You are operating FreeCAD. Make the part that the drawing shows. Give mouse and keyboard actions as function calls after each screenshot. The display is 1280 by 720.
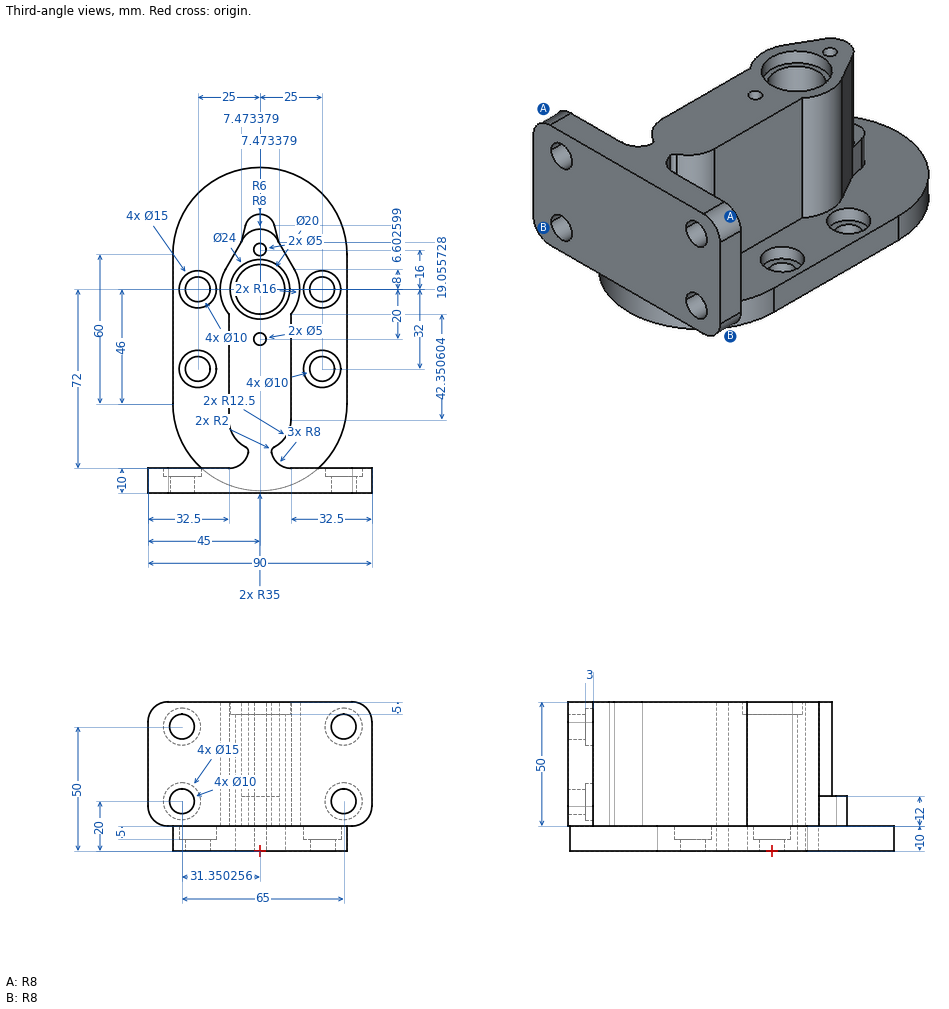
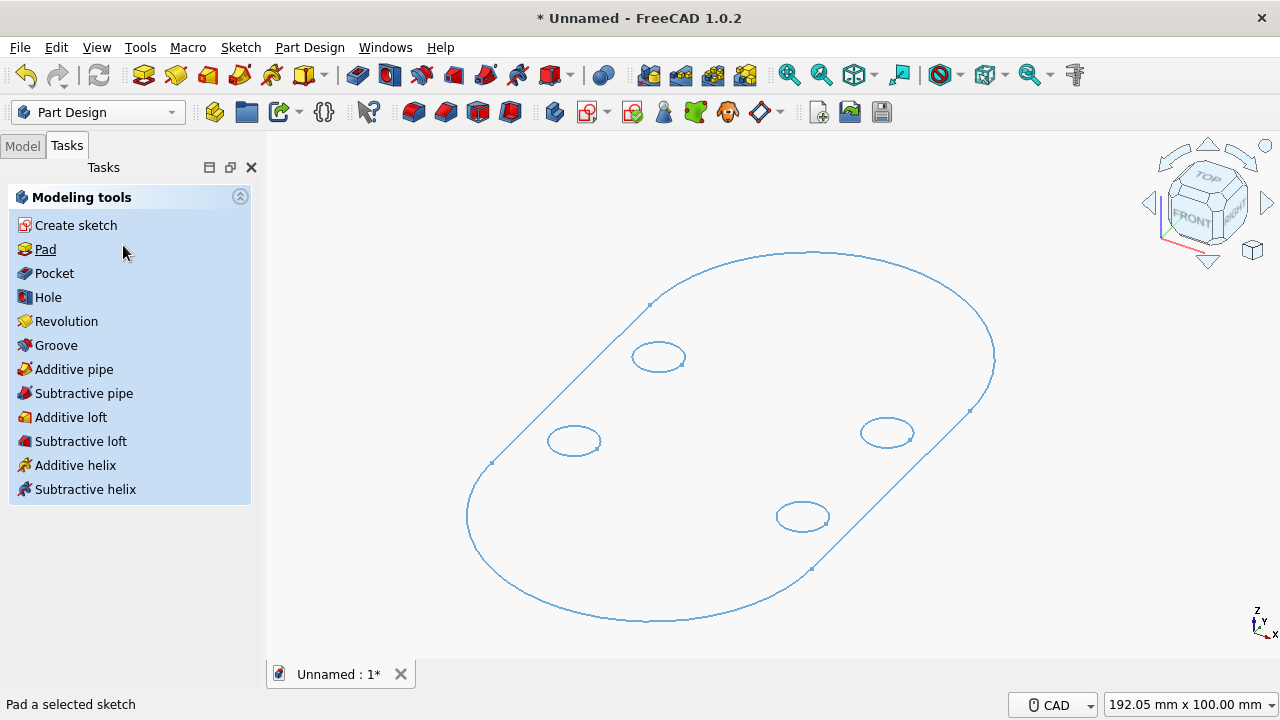
click(144, 76)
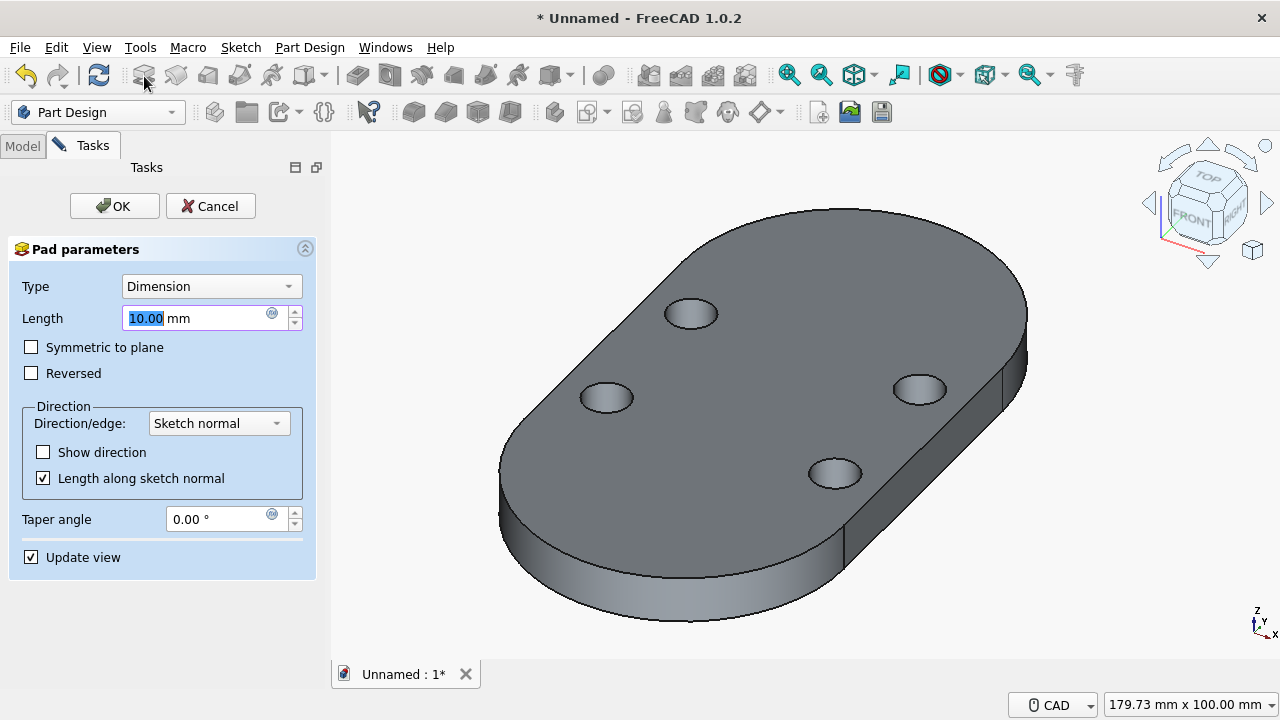
text(10)
key(Tab)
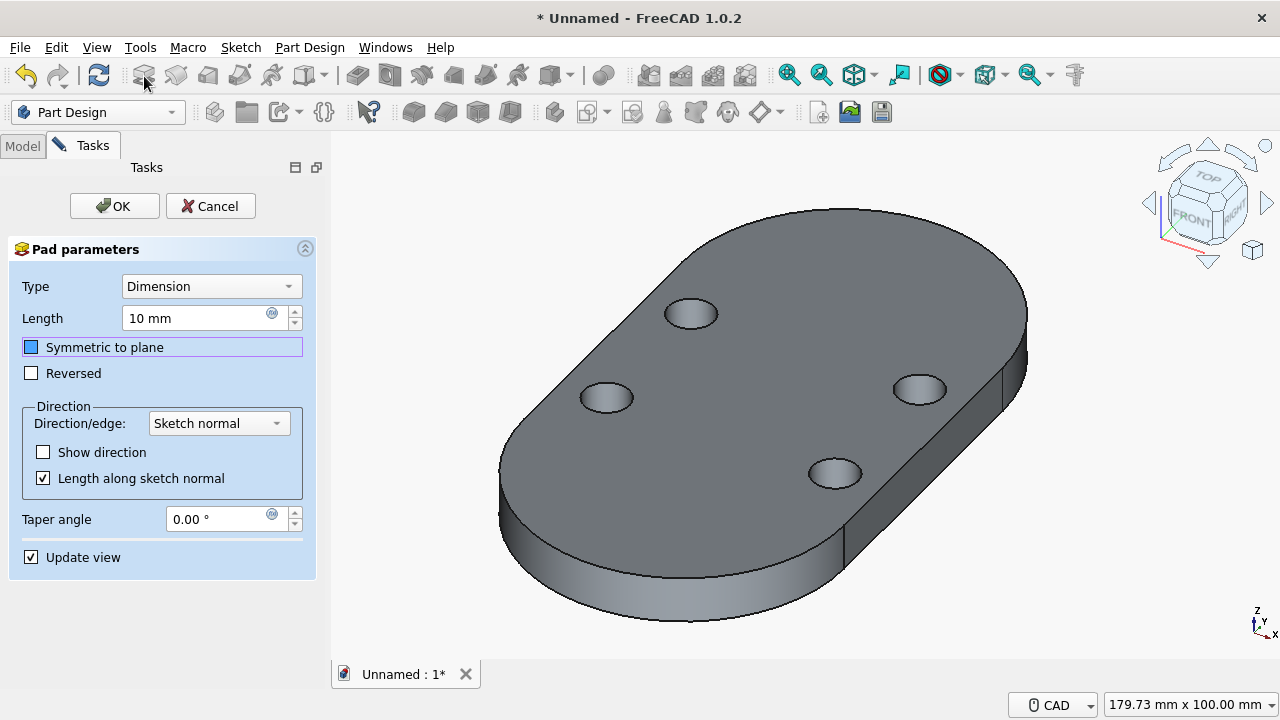
click(115, 206)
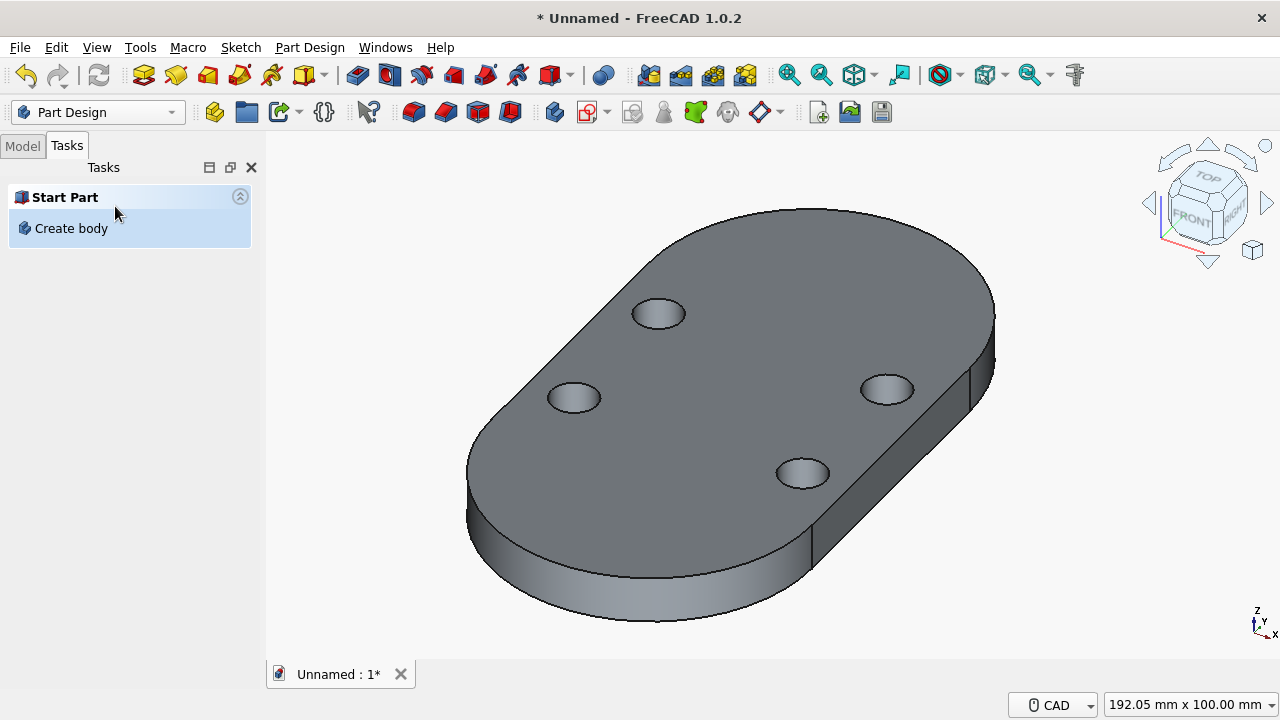
click(23, 145)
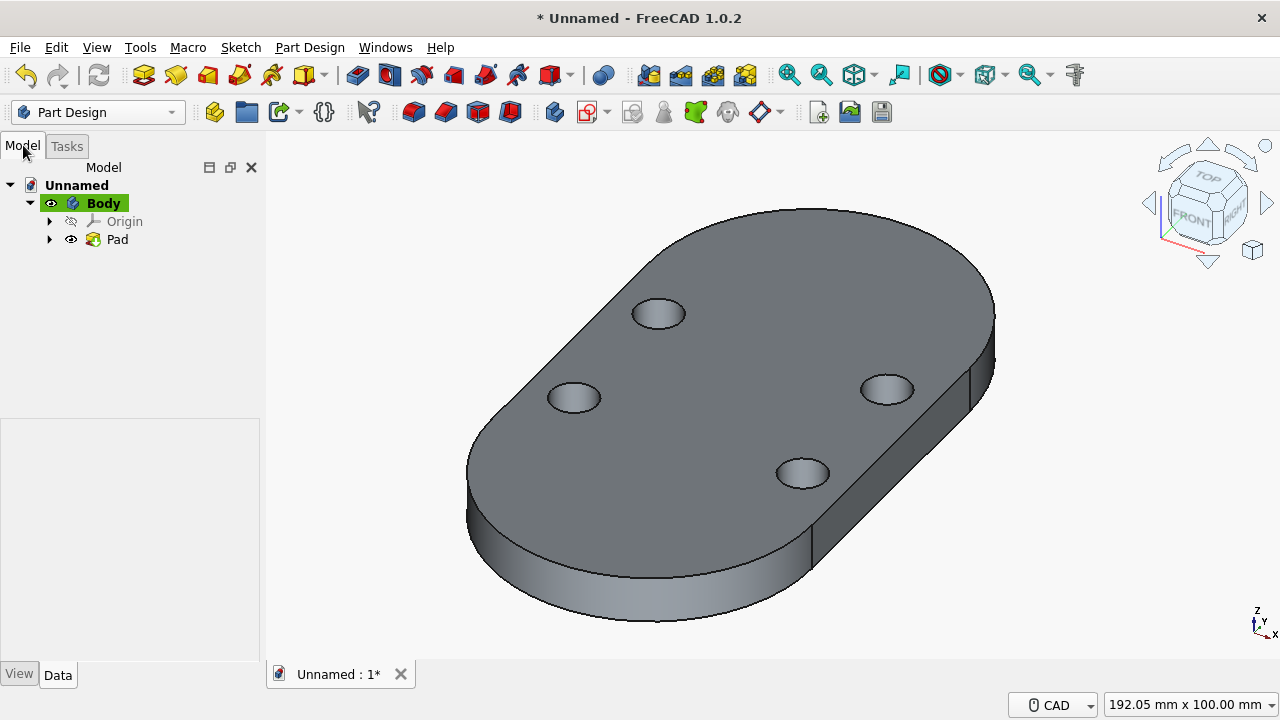
click(50, 221)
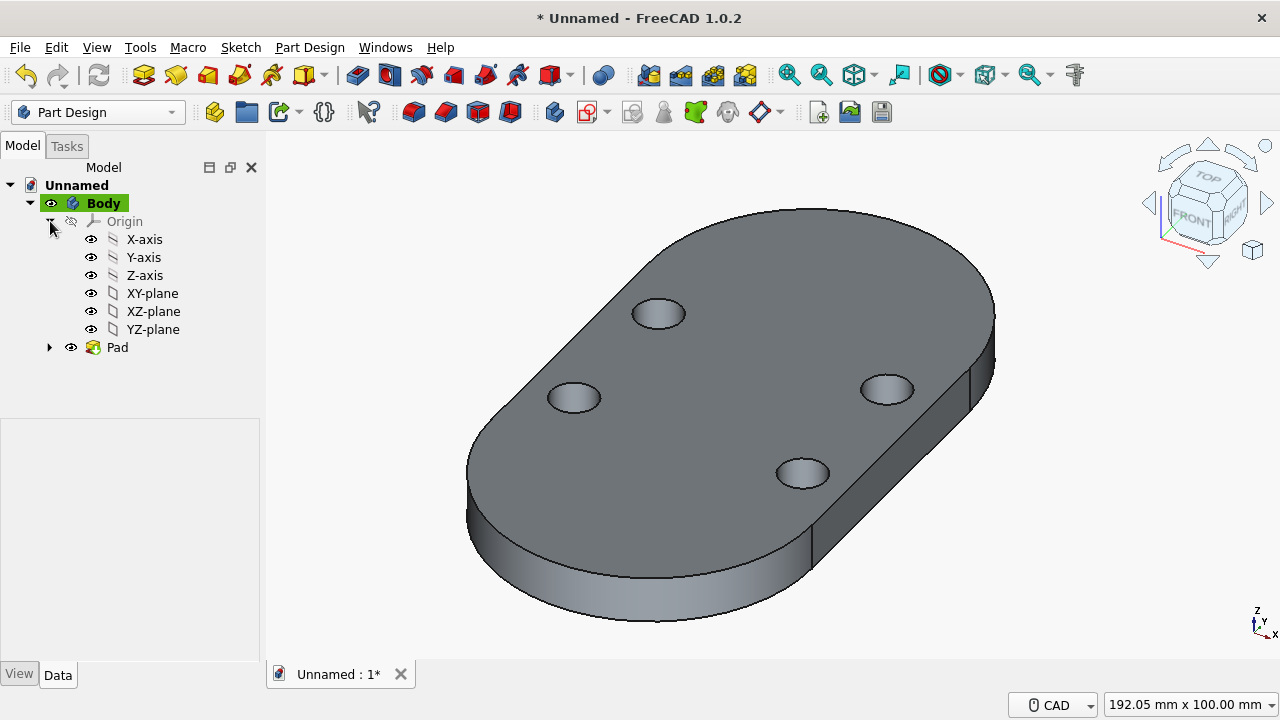
click(136, 293)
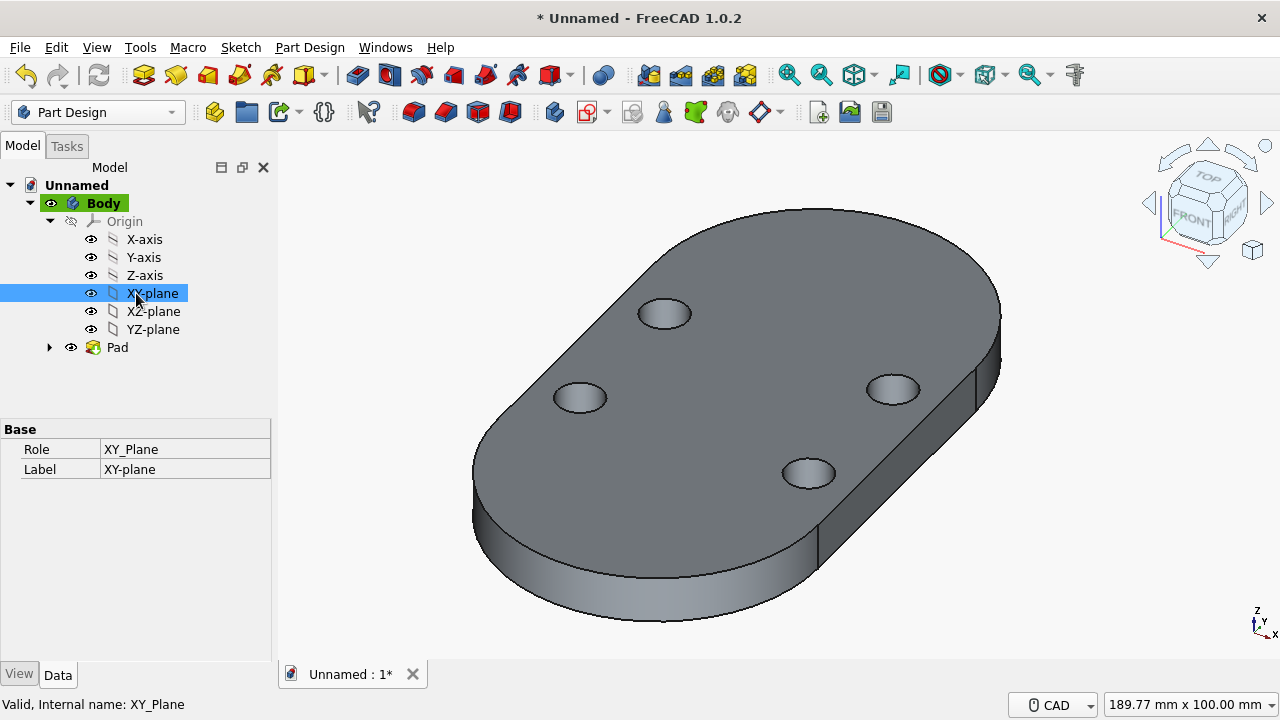
click(760, 112)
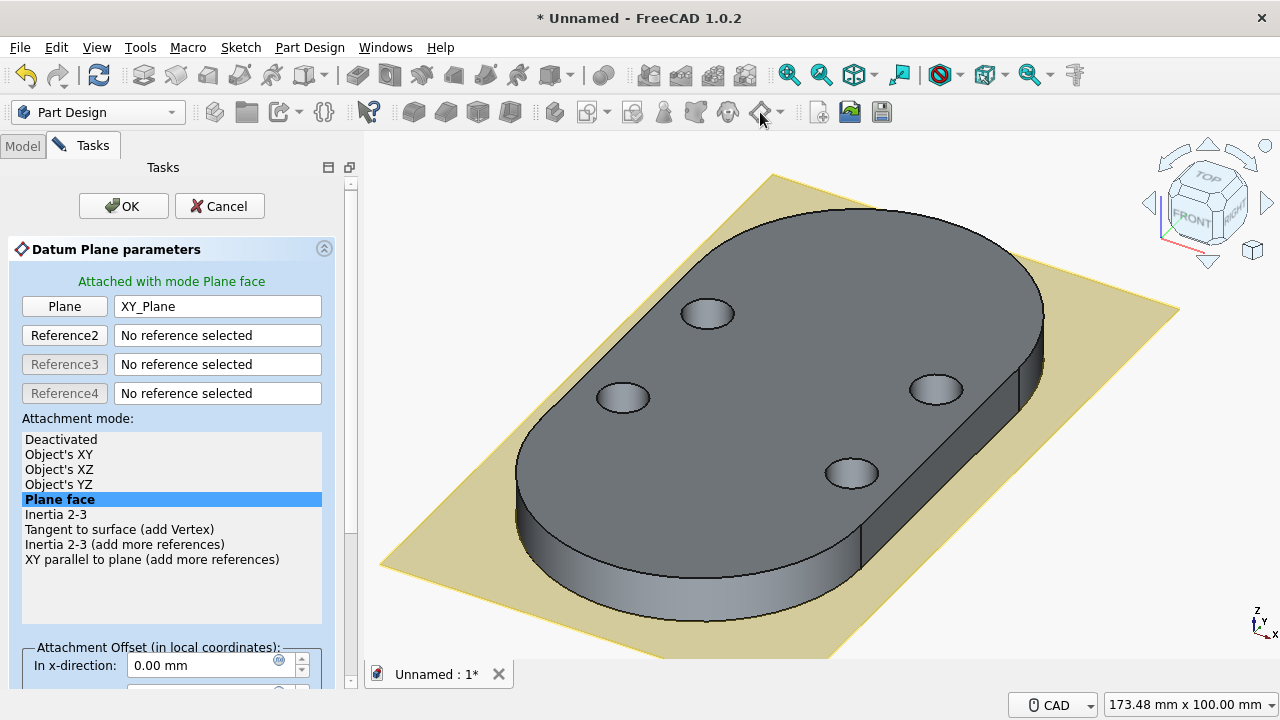
scroll(351, 432, down, 2)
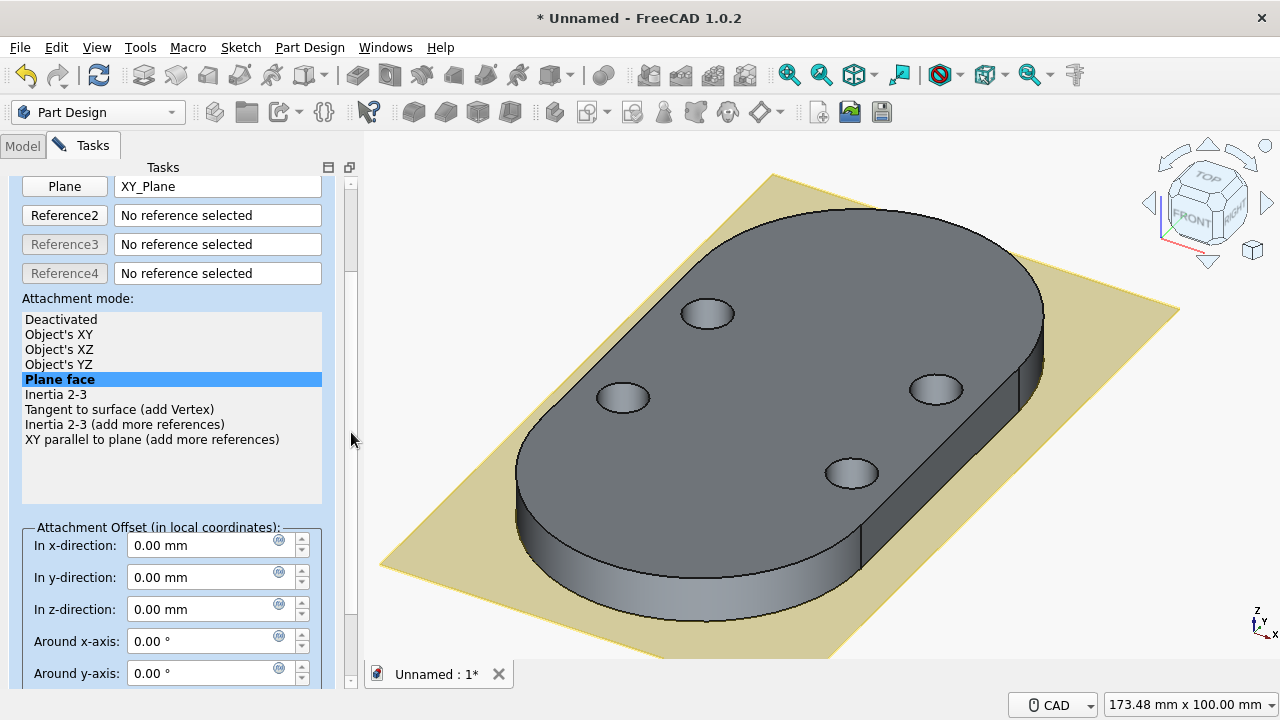
triple_click(210, 609)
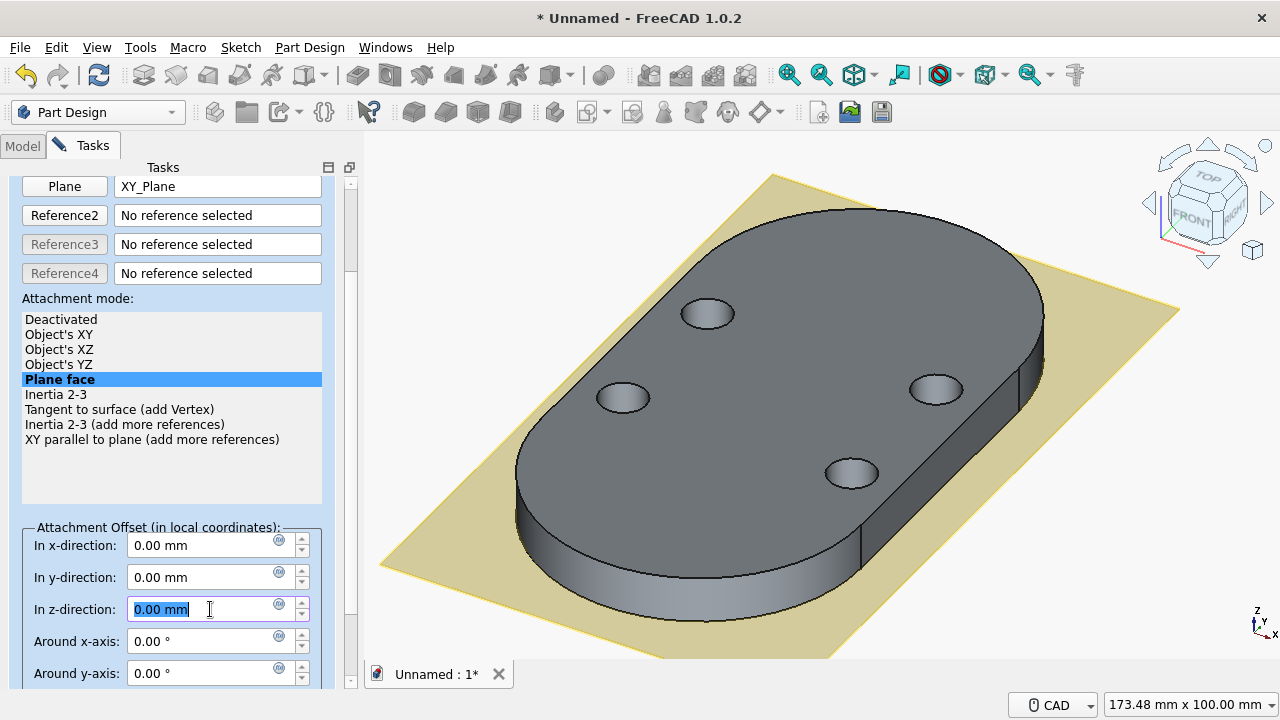
text(5)
key(Tab)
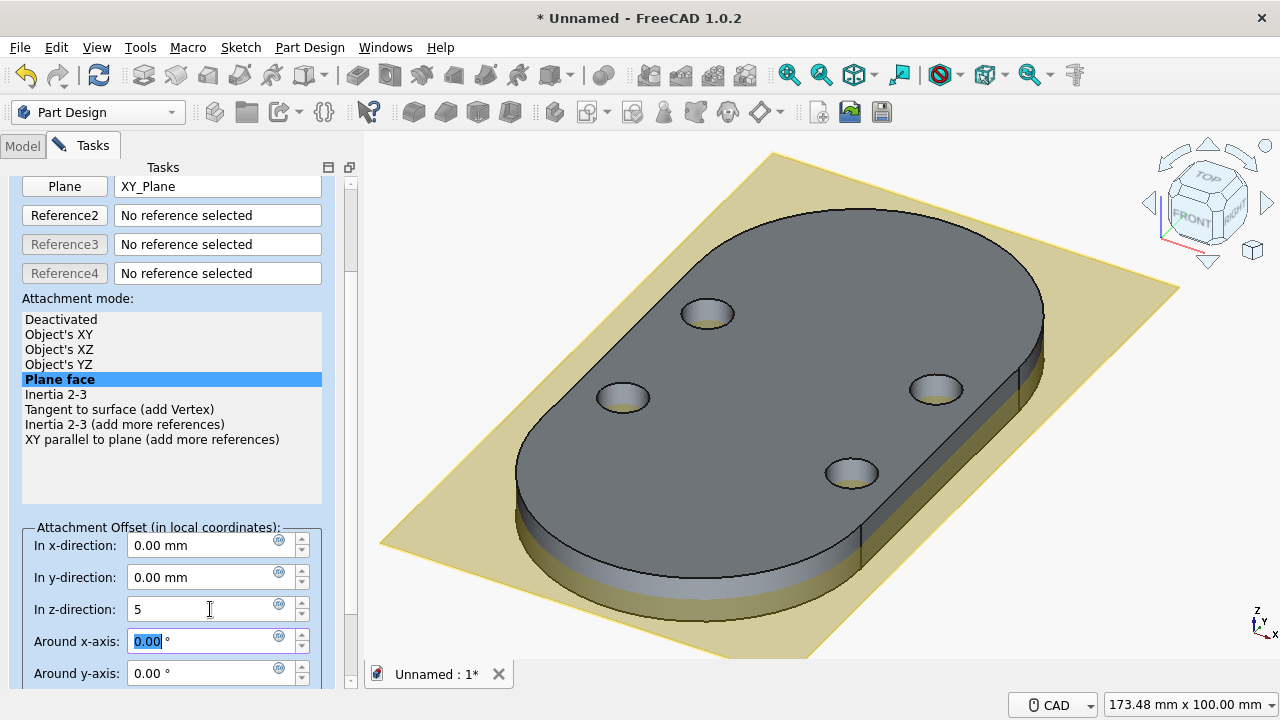
scroll(351, 432, up, 3)